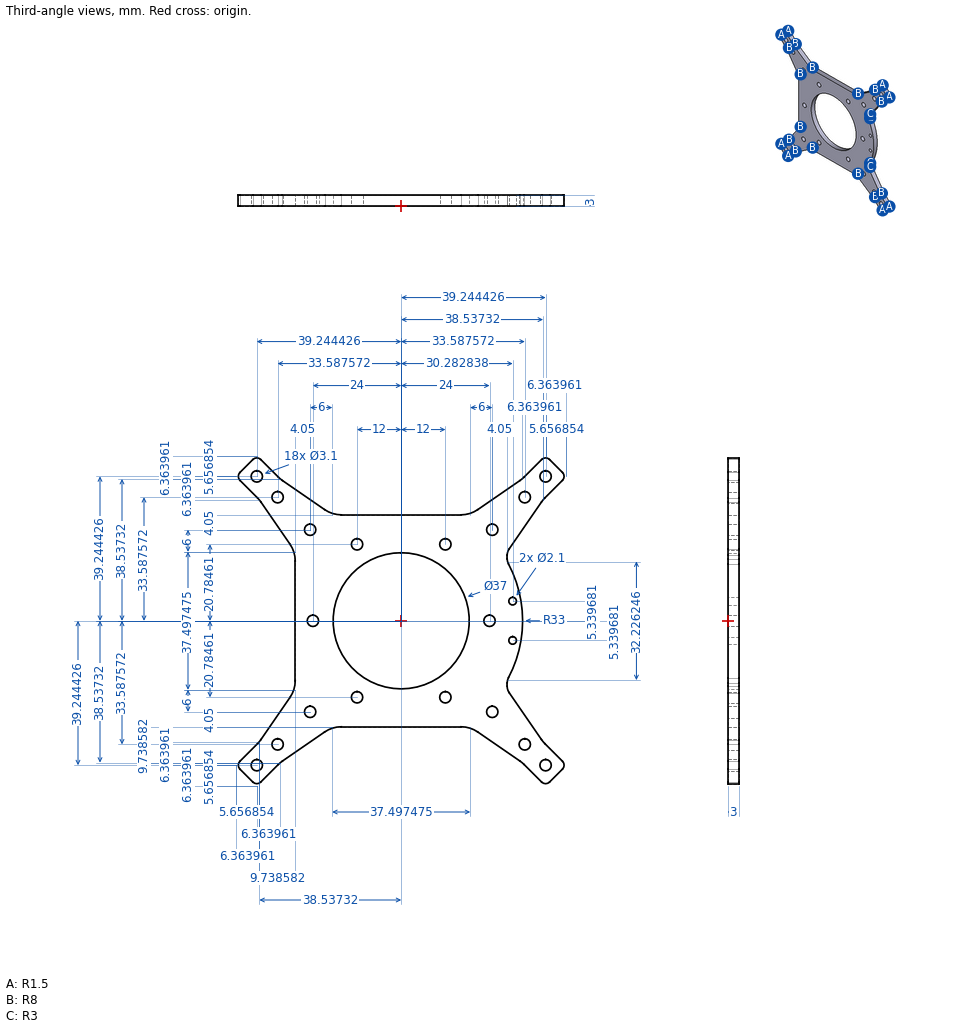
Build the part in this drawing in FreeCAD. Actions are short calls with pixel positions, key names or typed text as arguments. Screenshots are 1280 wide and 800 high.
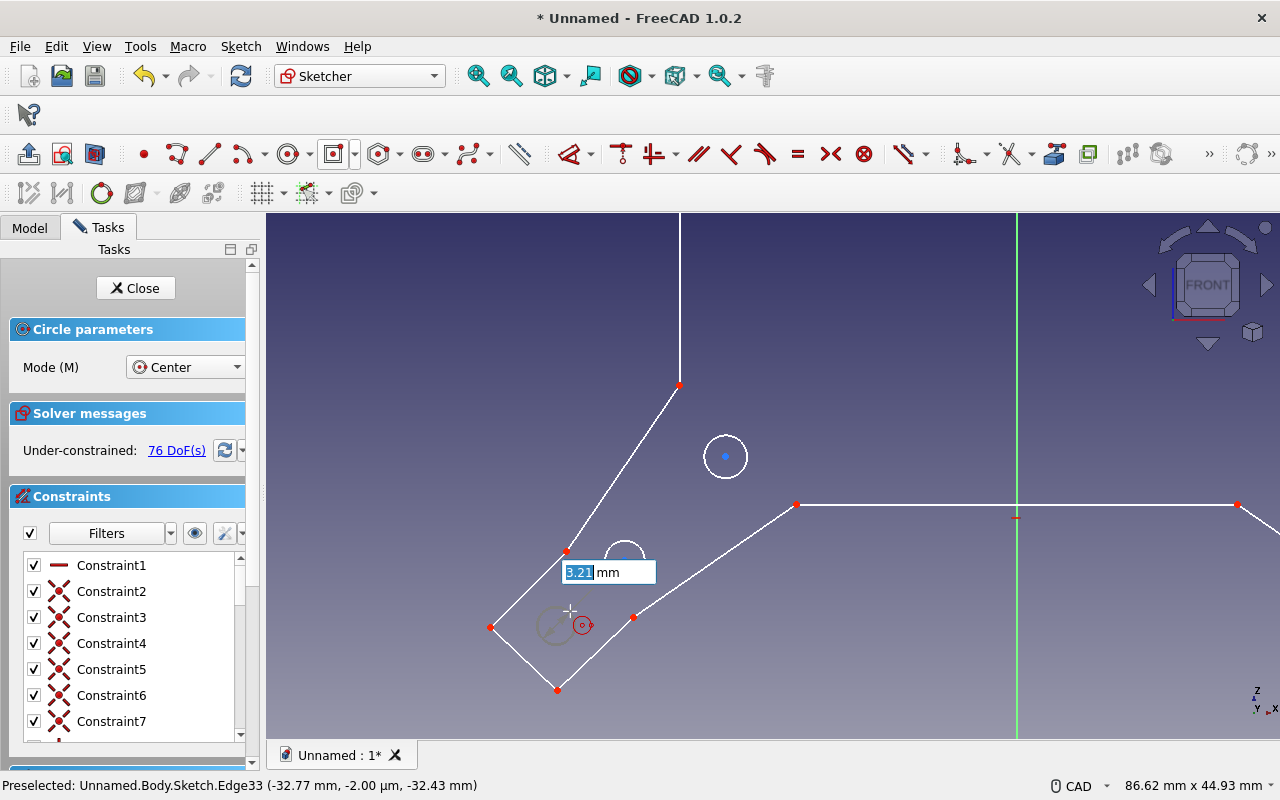
click(570, 610)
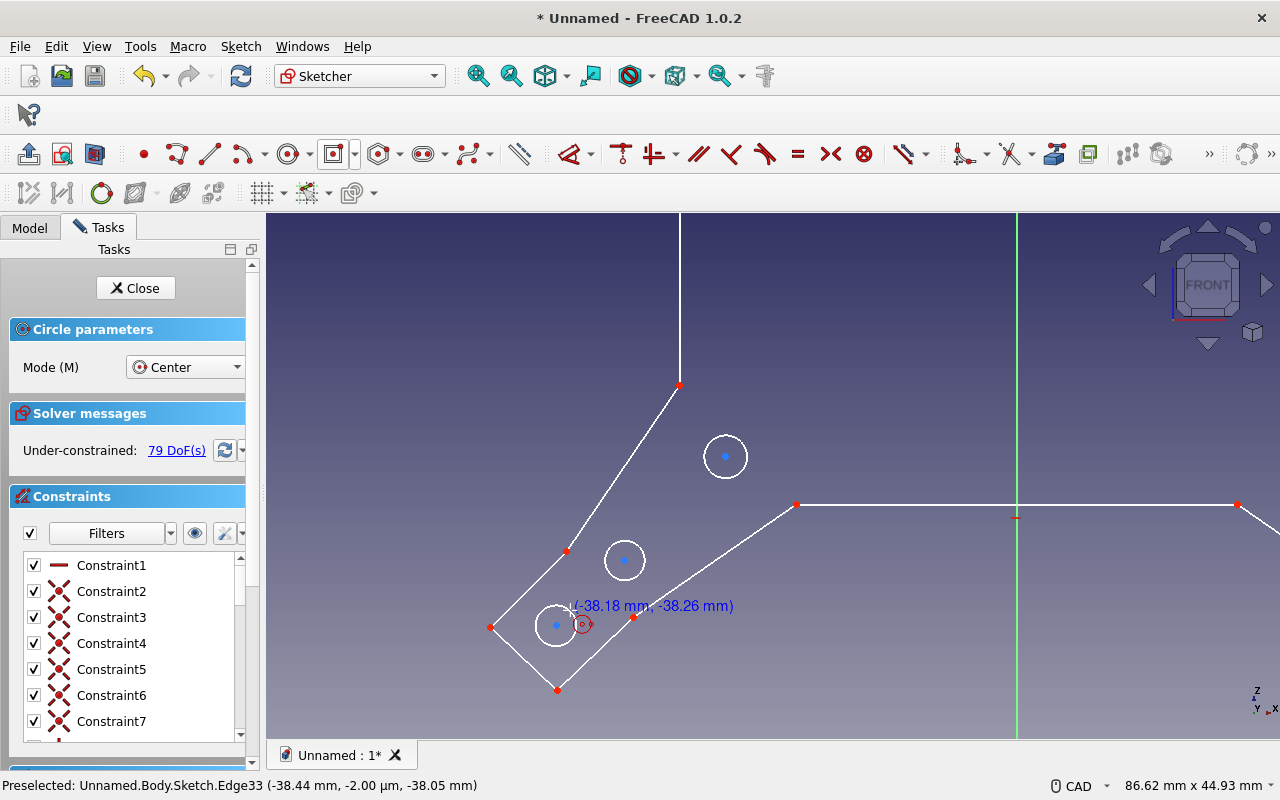
scroll(876, 406, up, 2)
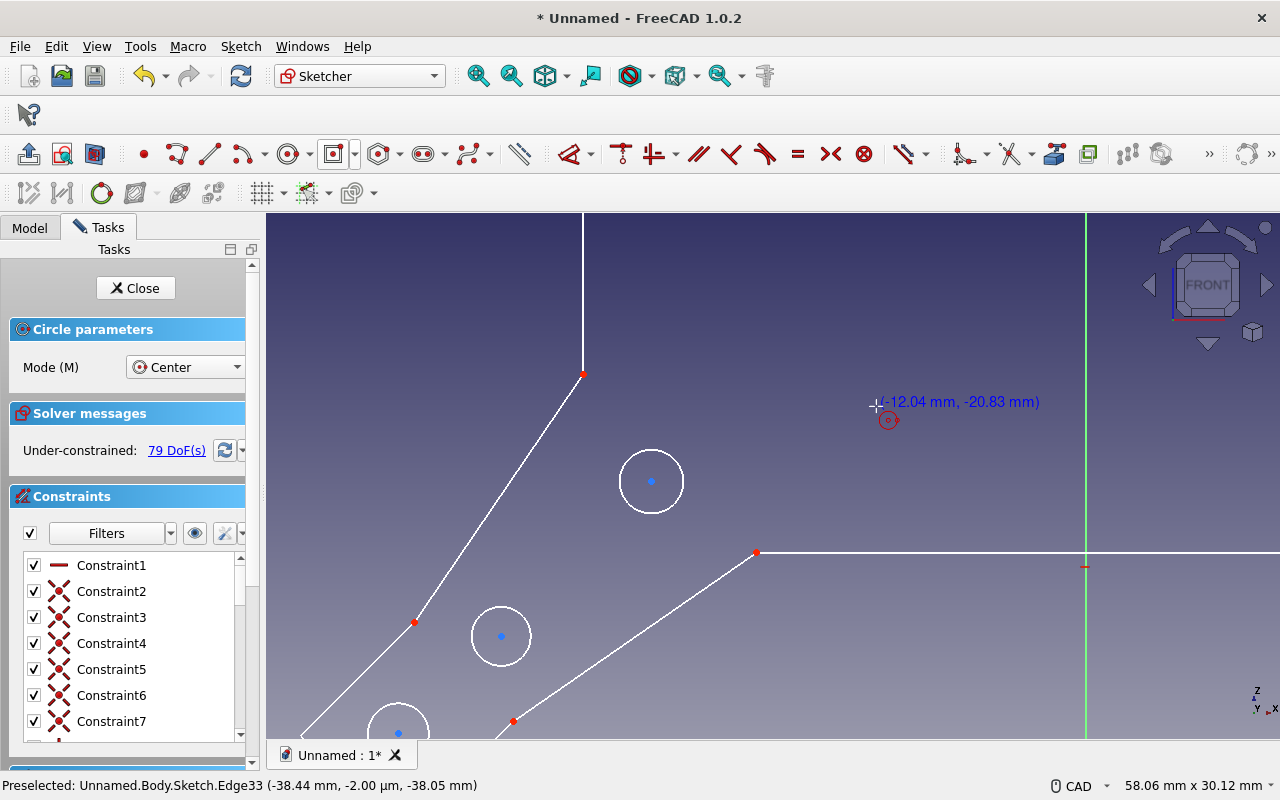
scroll(608, 585, down, 8)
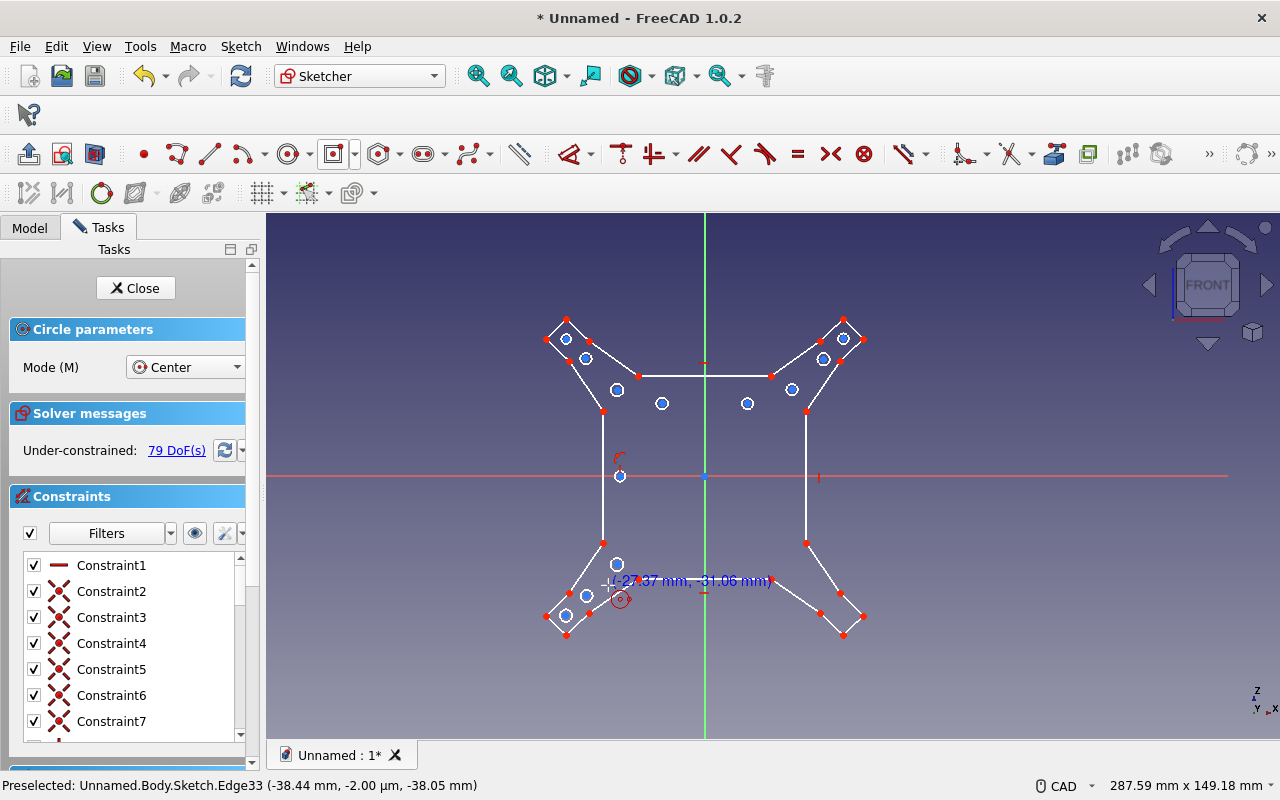
click(662, 550)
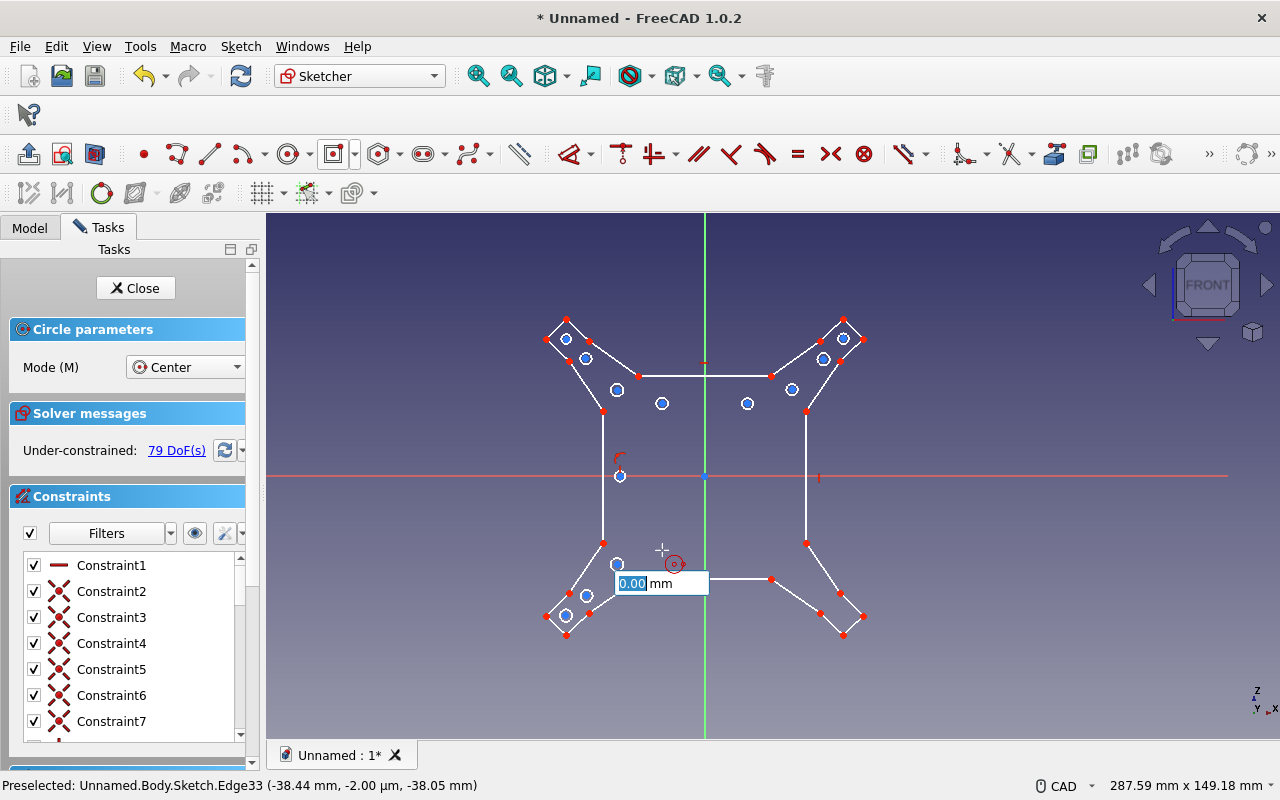
scroll(666, 546, up, 6)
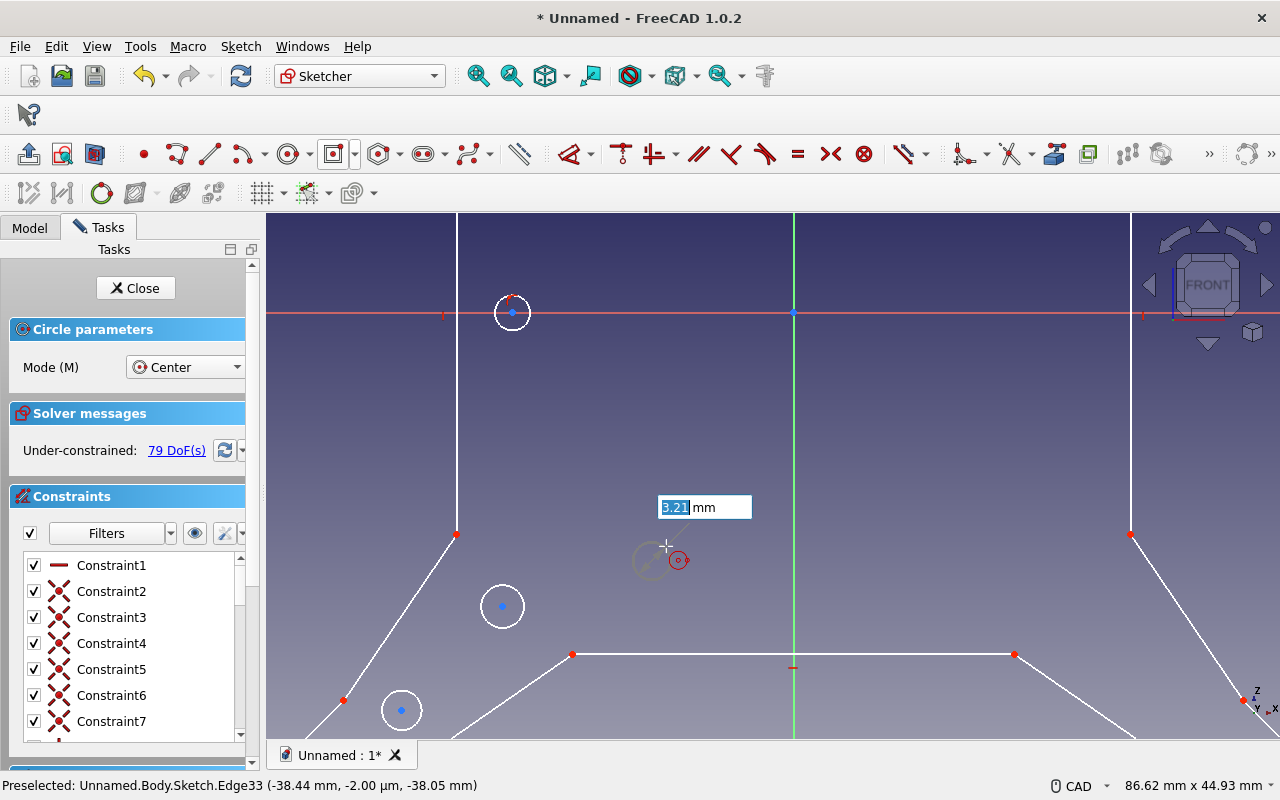
click(666, 543)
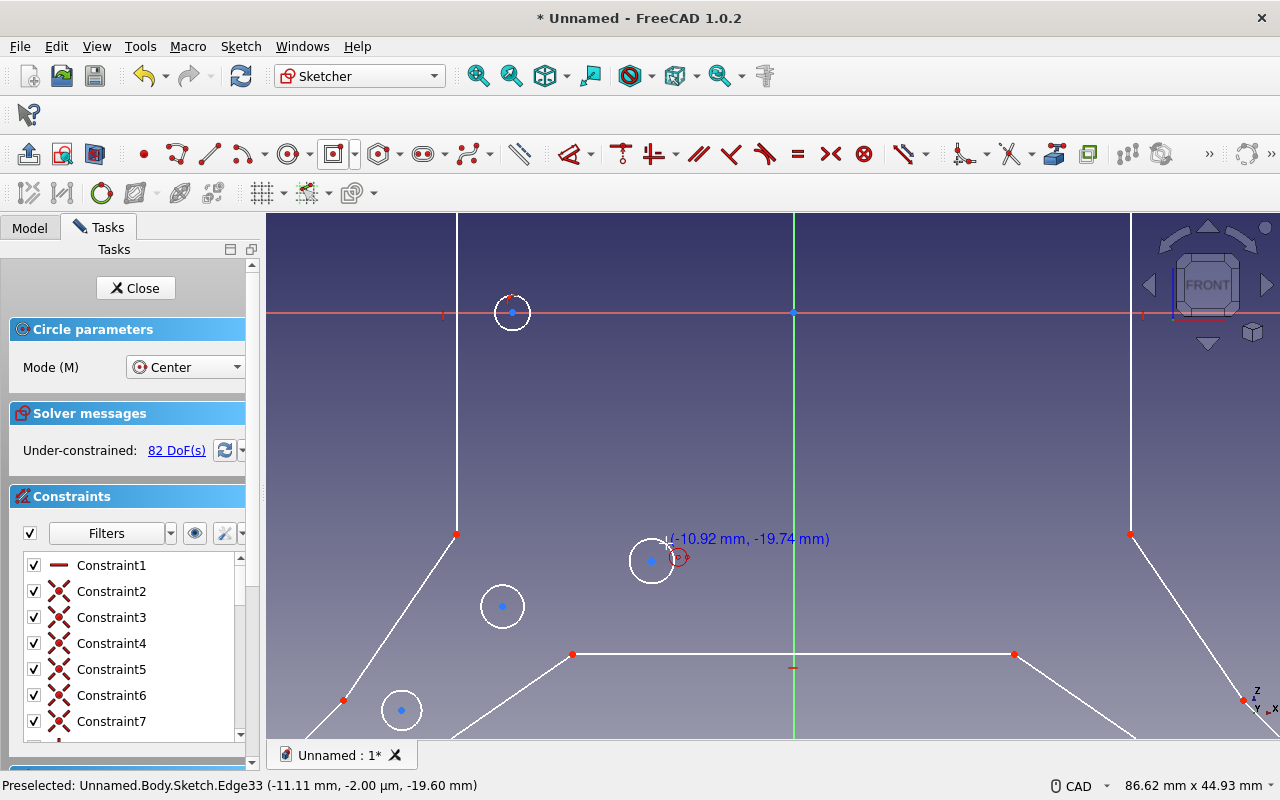
click(794, 313)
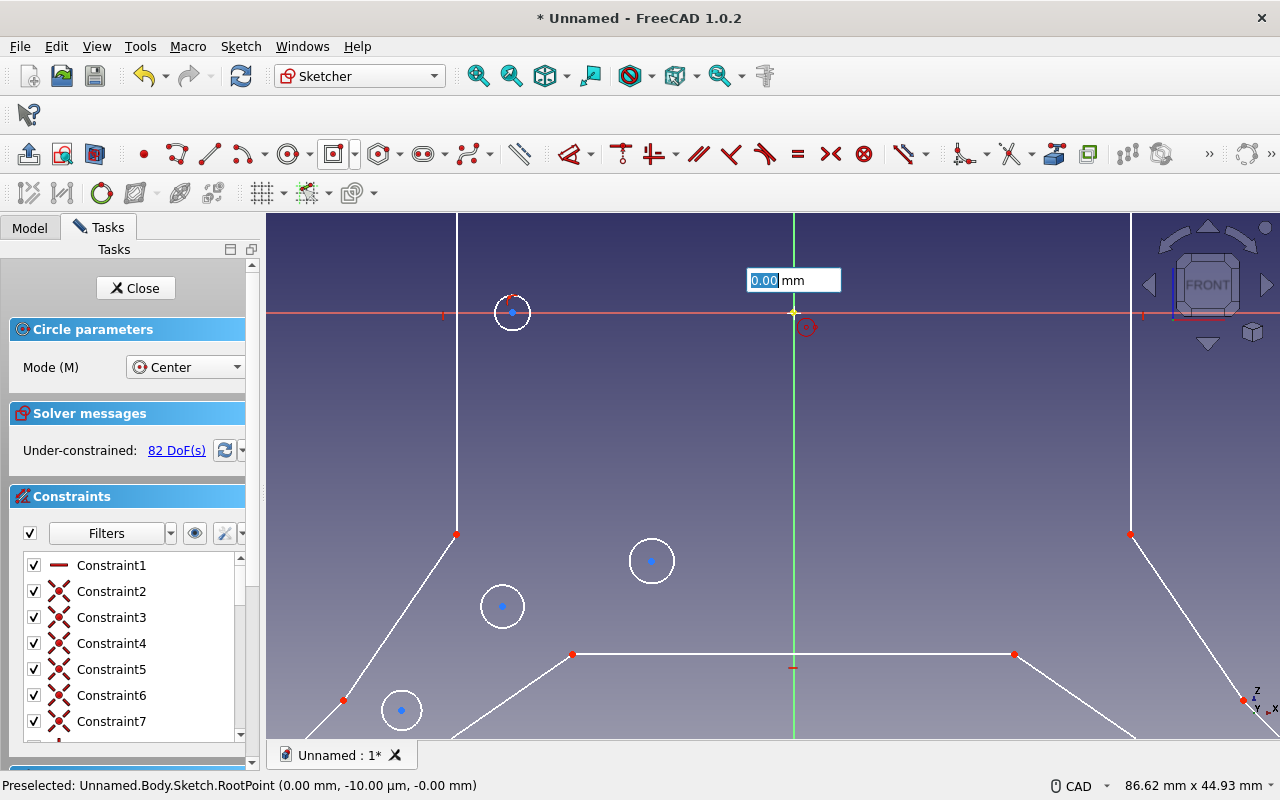
scroll(666, 546, down, 6)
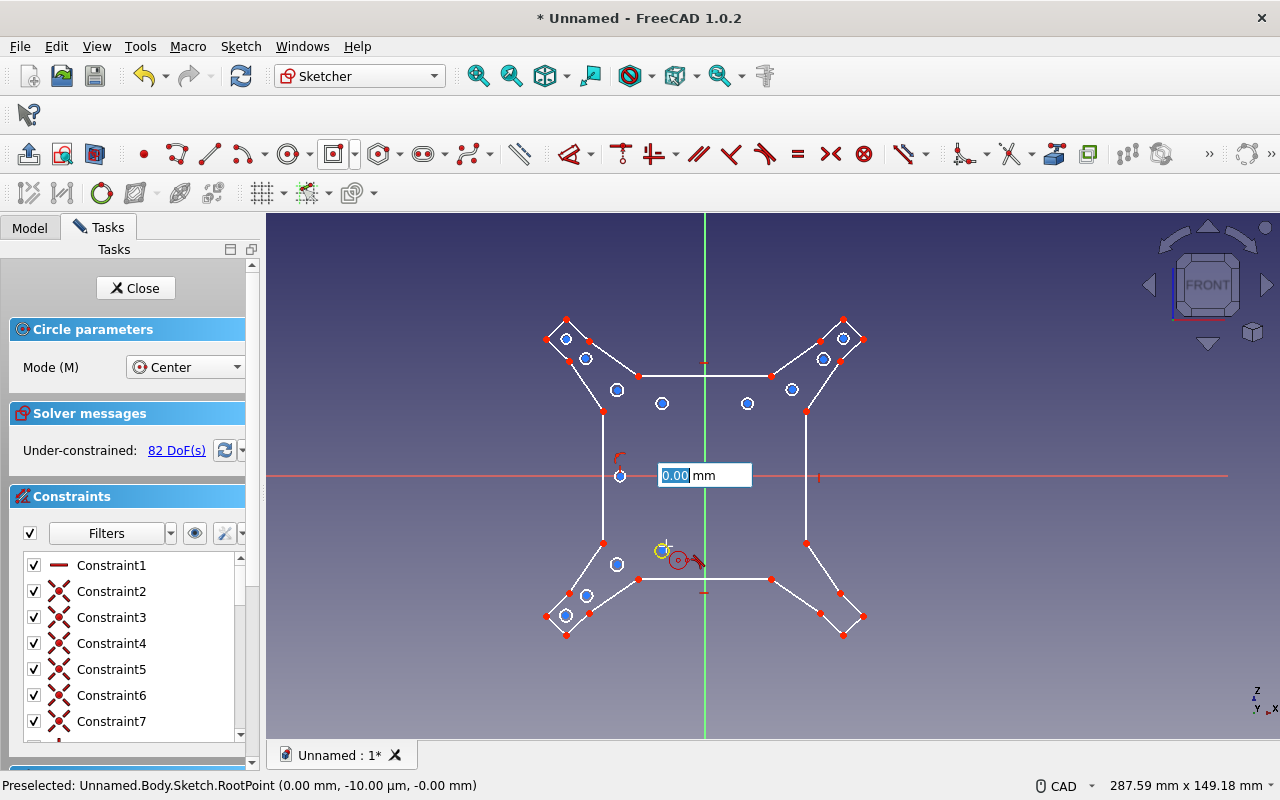
click(751, 430)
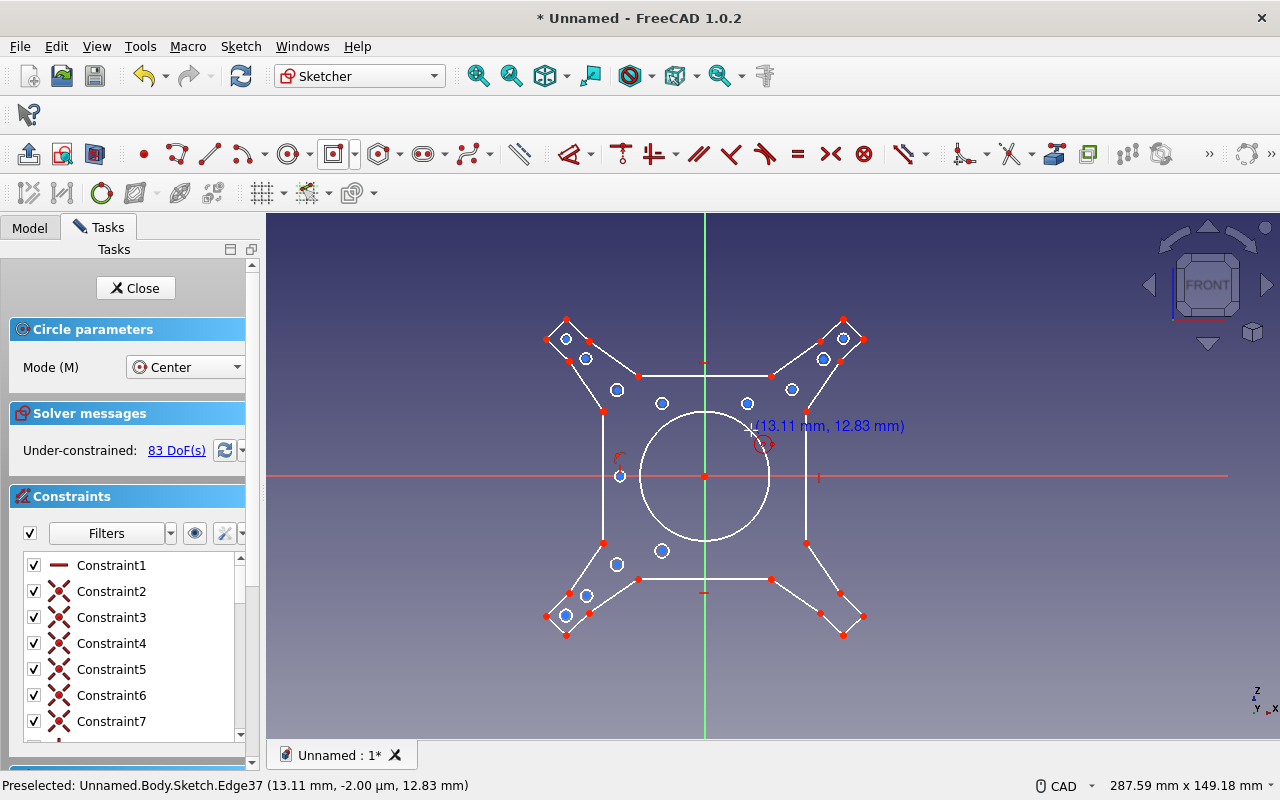
scroll(789, 476, up, 8)